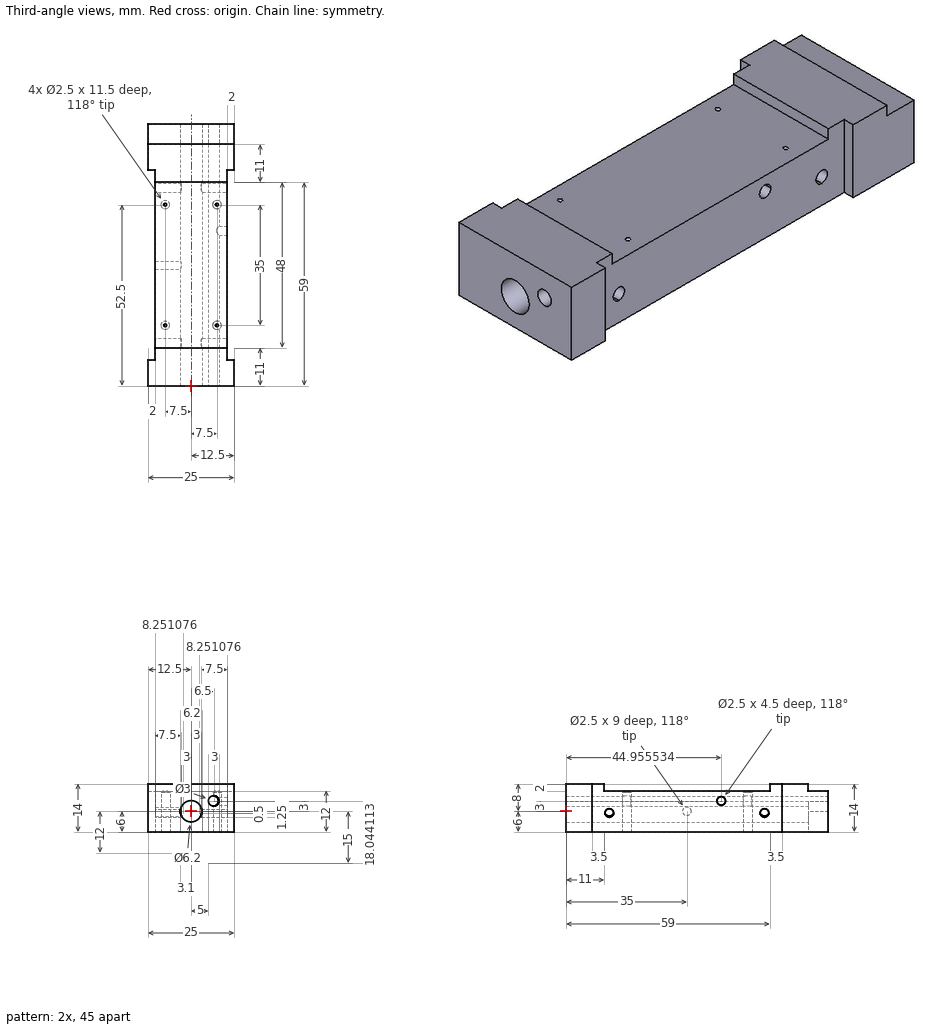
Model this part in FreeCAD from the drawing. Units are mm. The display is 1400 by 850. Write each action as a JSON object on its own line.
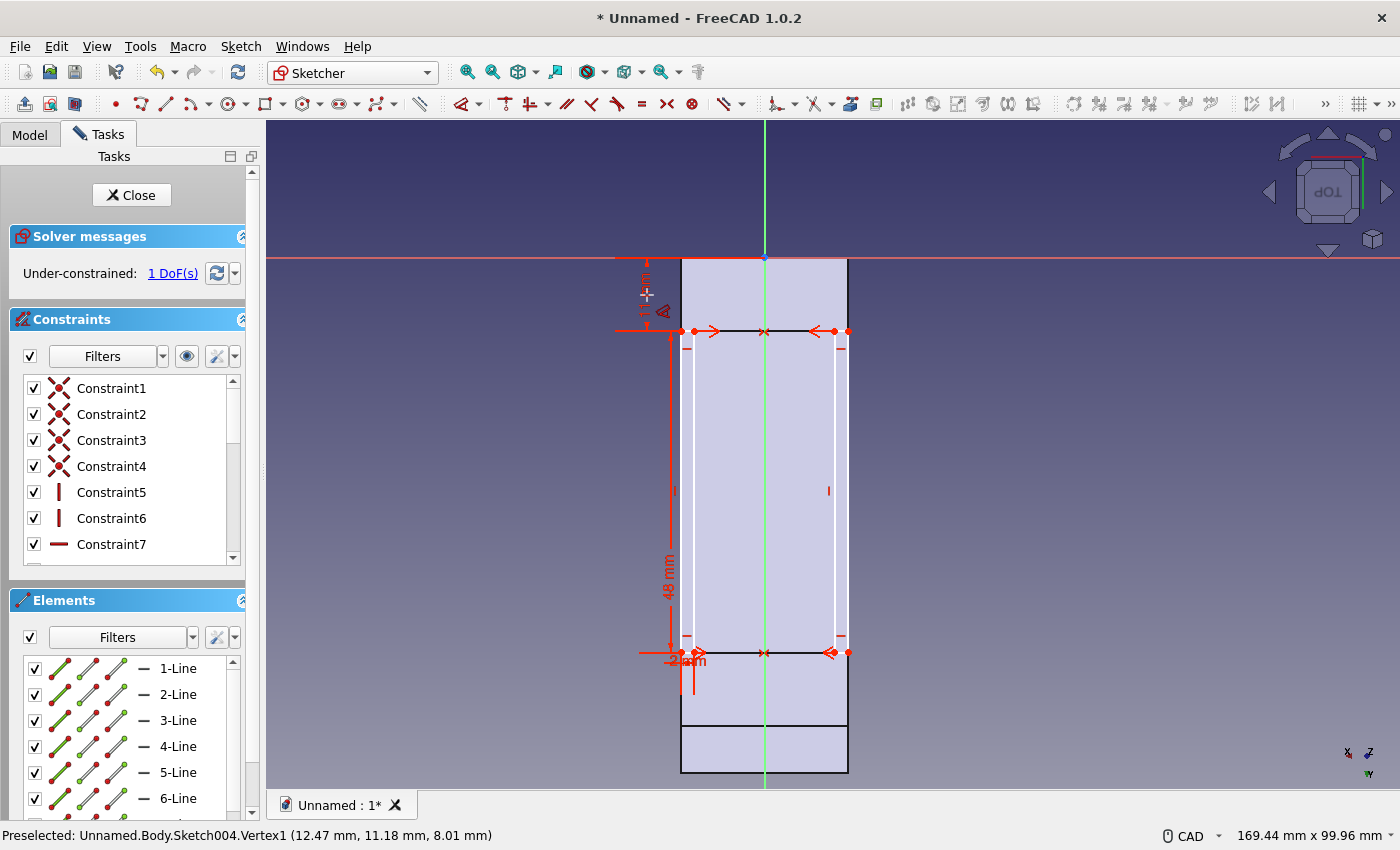
{"action": "left_click", "coordinate": [681, 331]}
{"action": "left_click", "coordinate": [723, 224]}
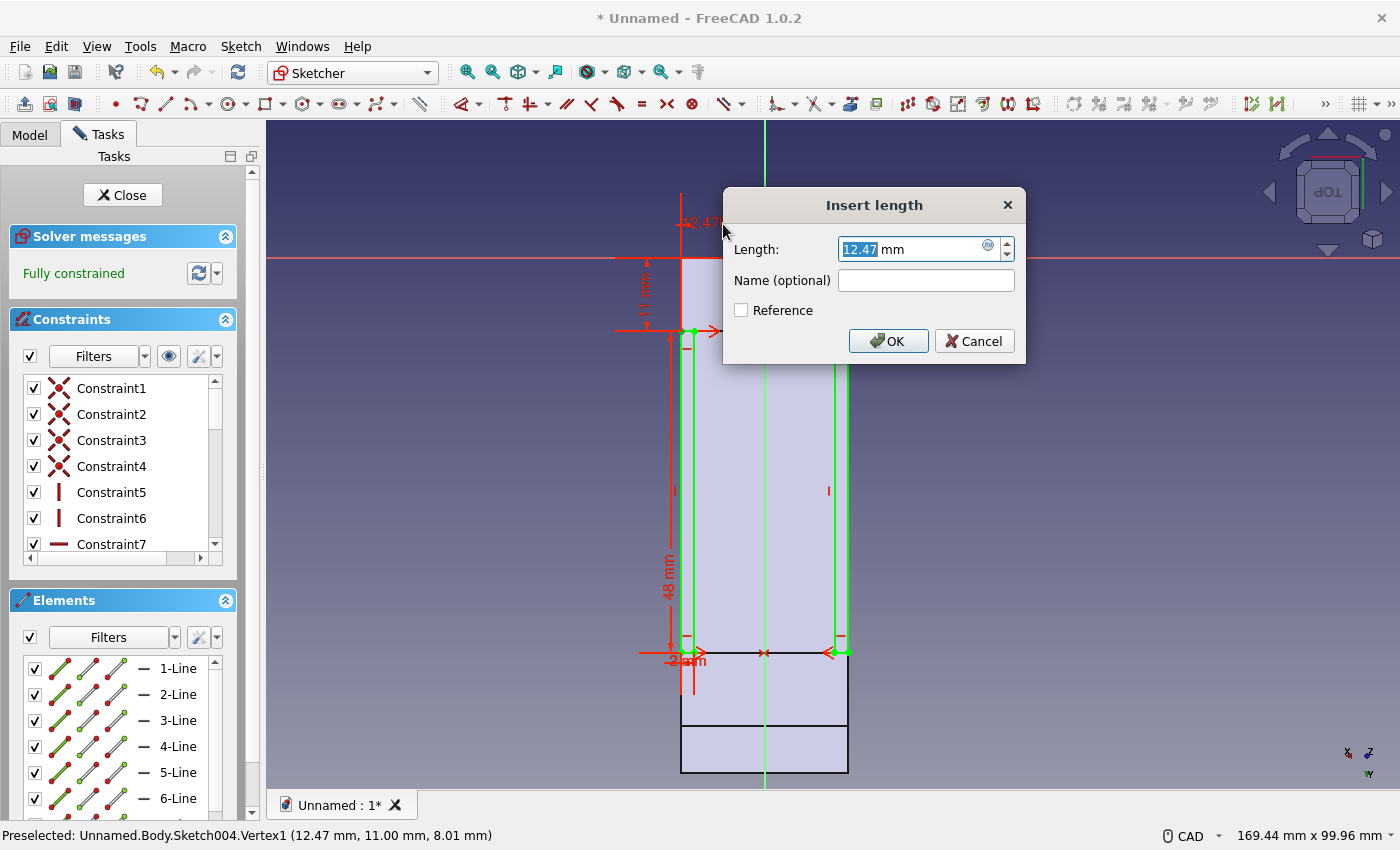
{"action": "type", "text": "12.5"}
{"action": "key", "text": "Return"}
{"action": "key", "text": "Escape"}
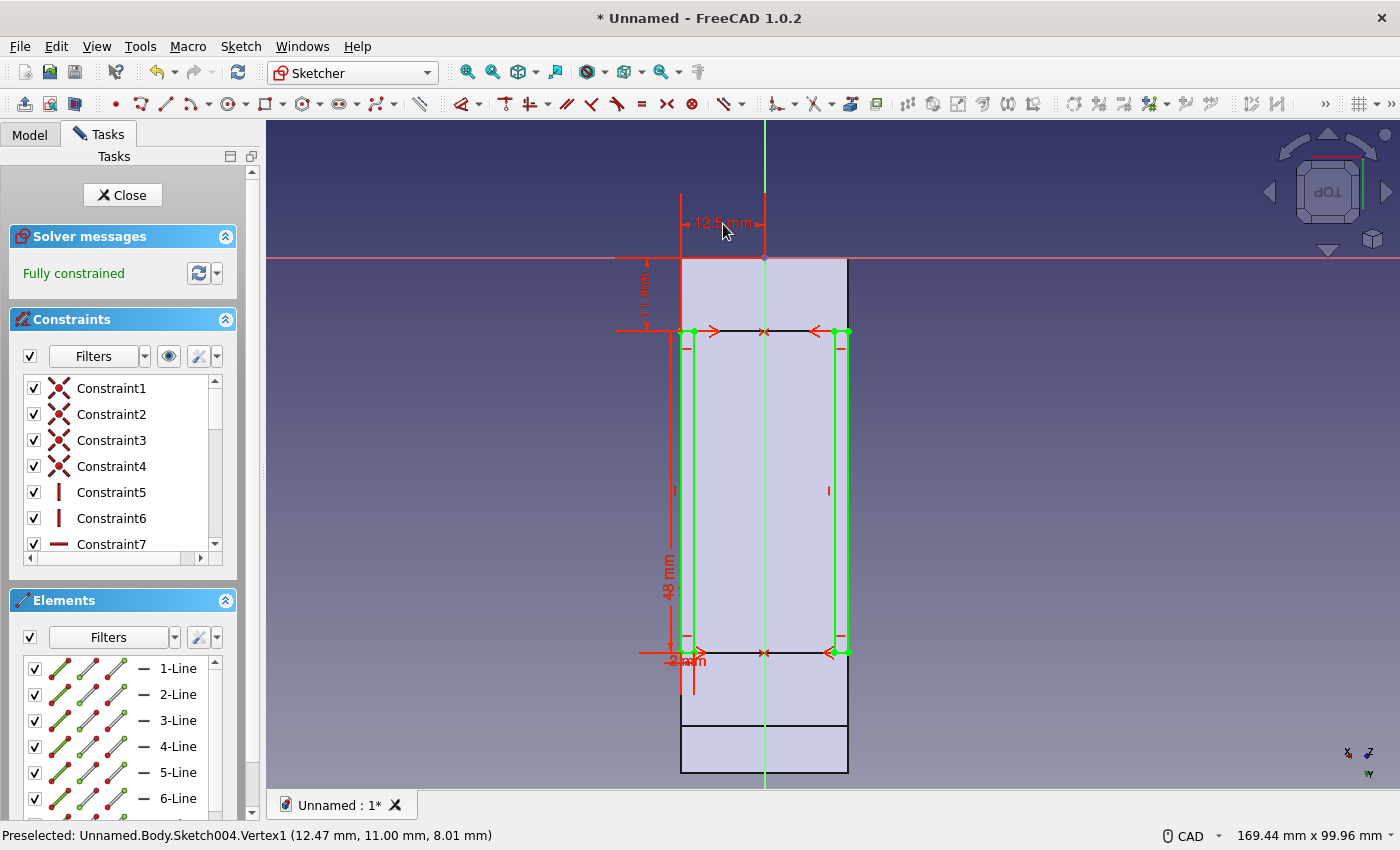
{"action": "left_click", "coordinate": [123, 195]}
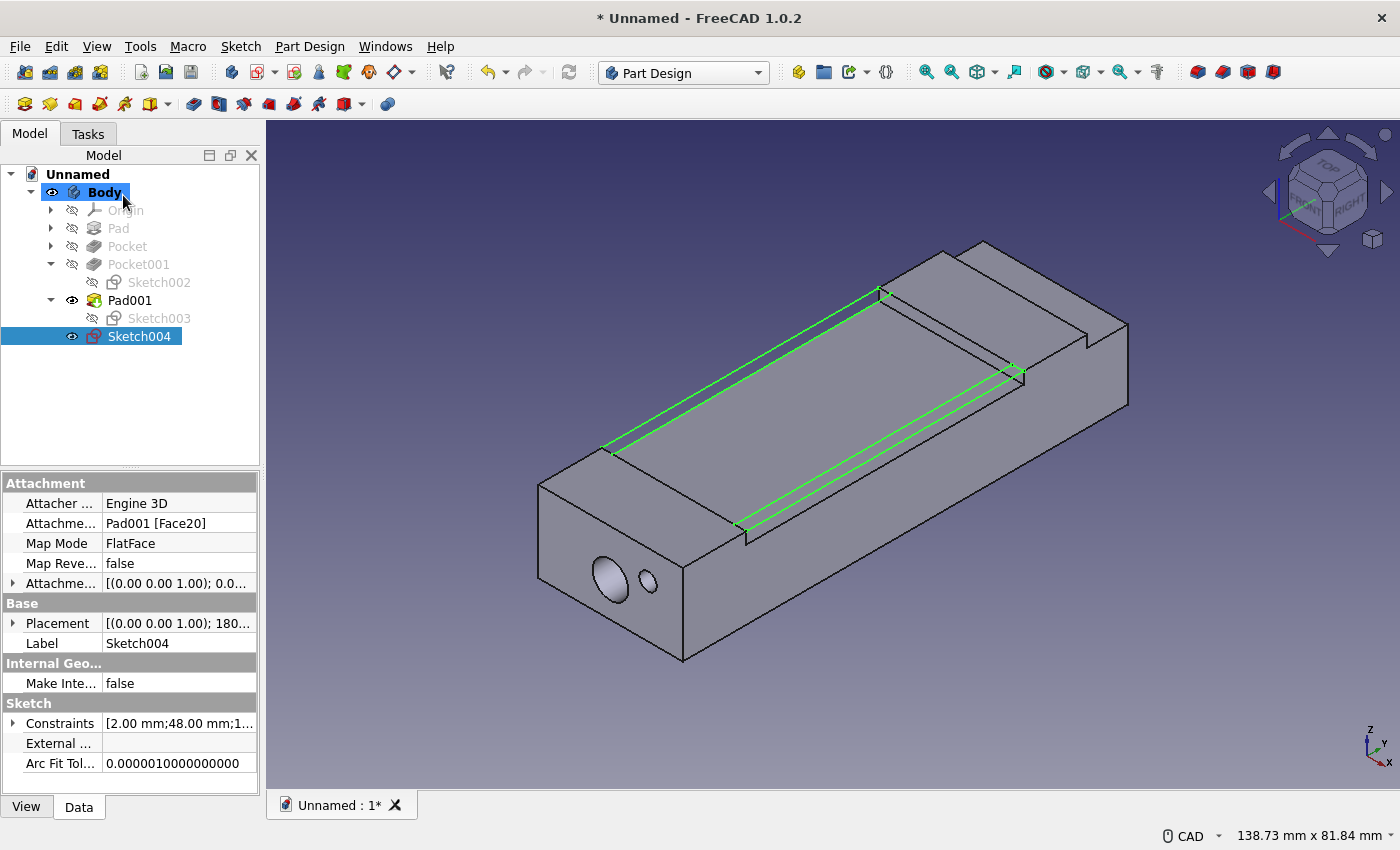
{"action": "left_click", "coordinate": [194, 104]}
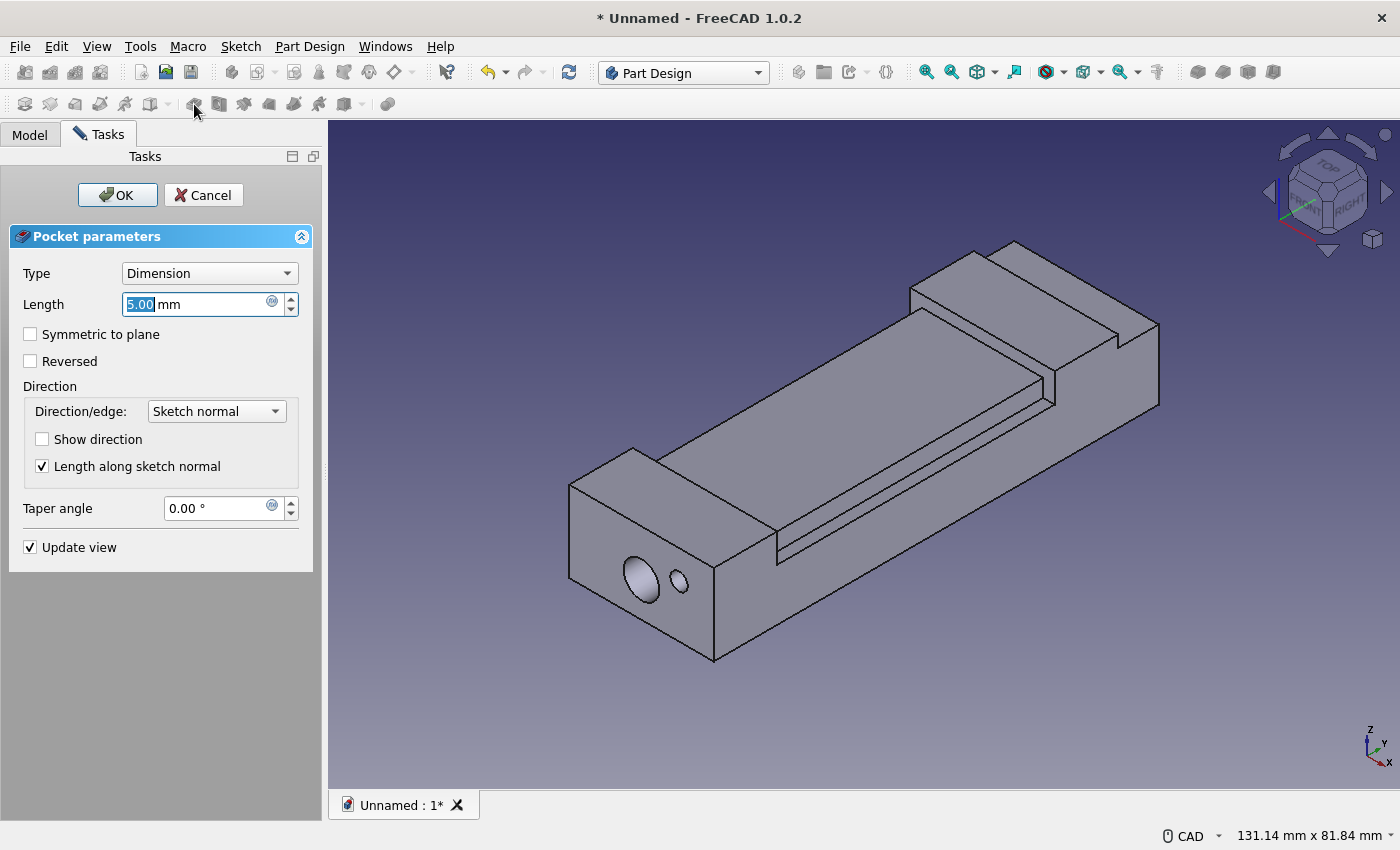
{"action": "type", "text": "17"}
{"action": "key", "text": "Tab"}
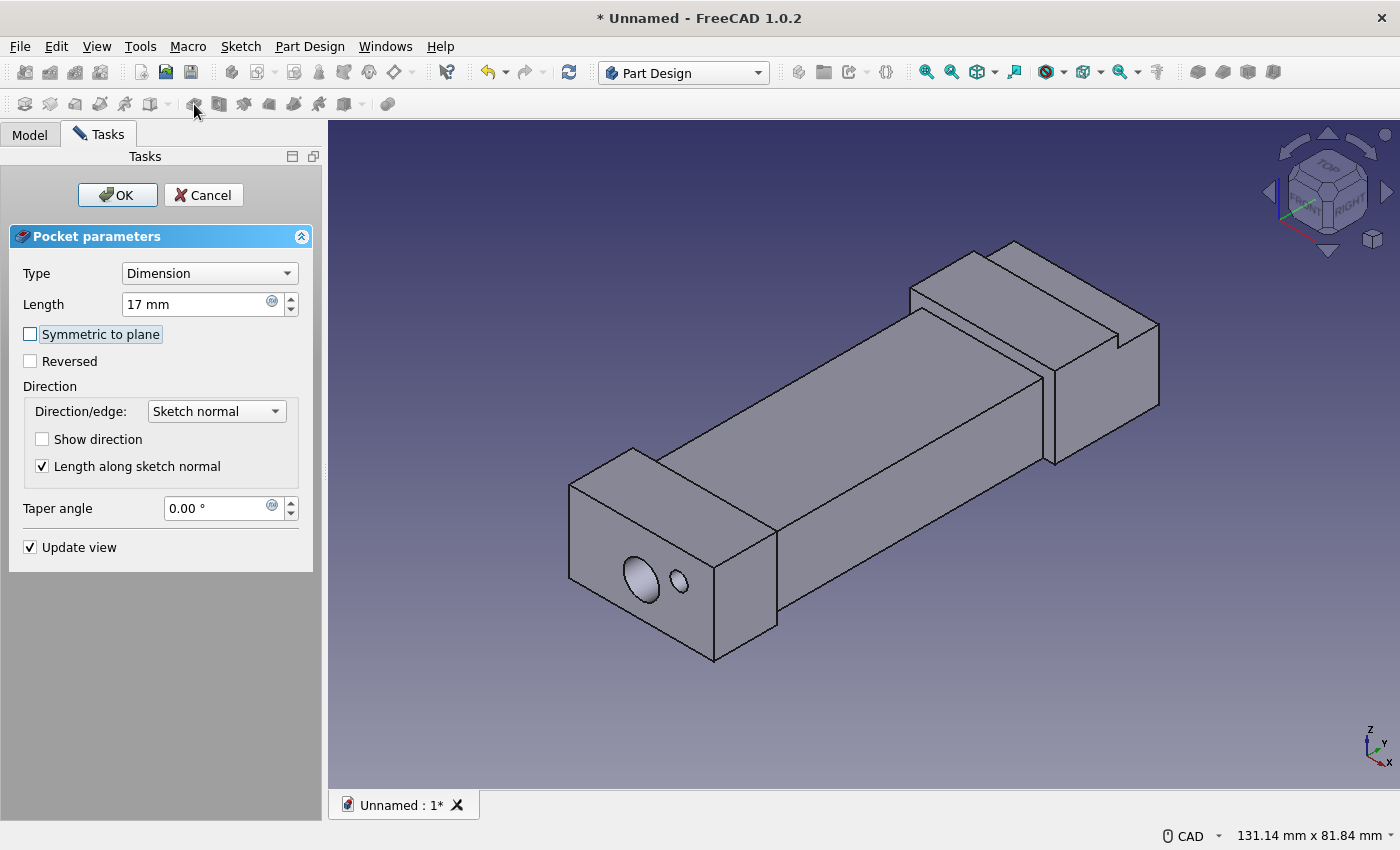
{"action": "left_click", "coordinate": [118, 195]}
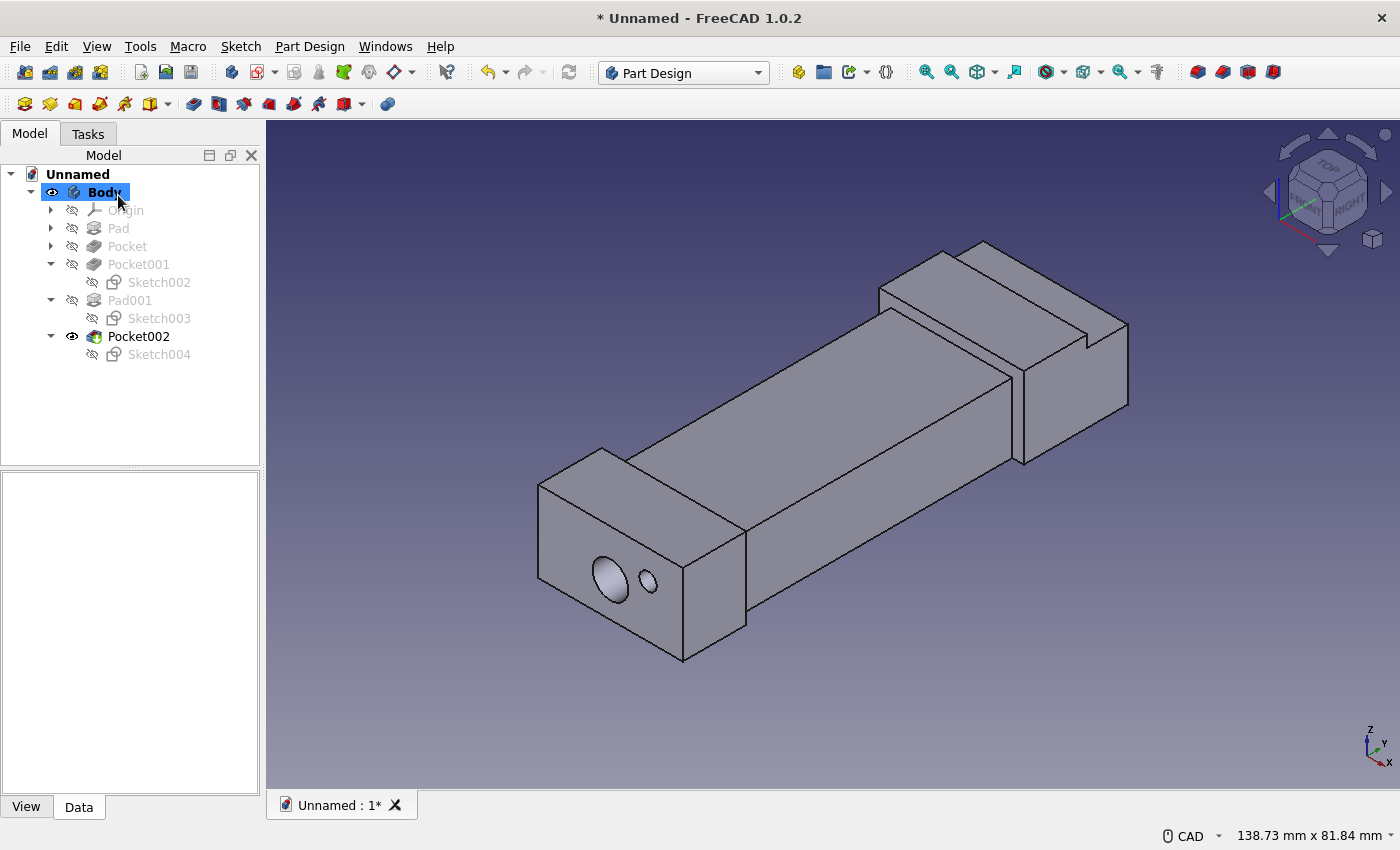
{"action": "left_click", "coordinate": [51, 210]}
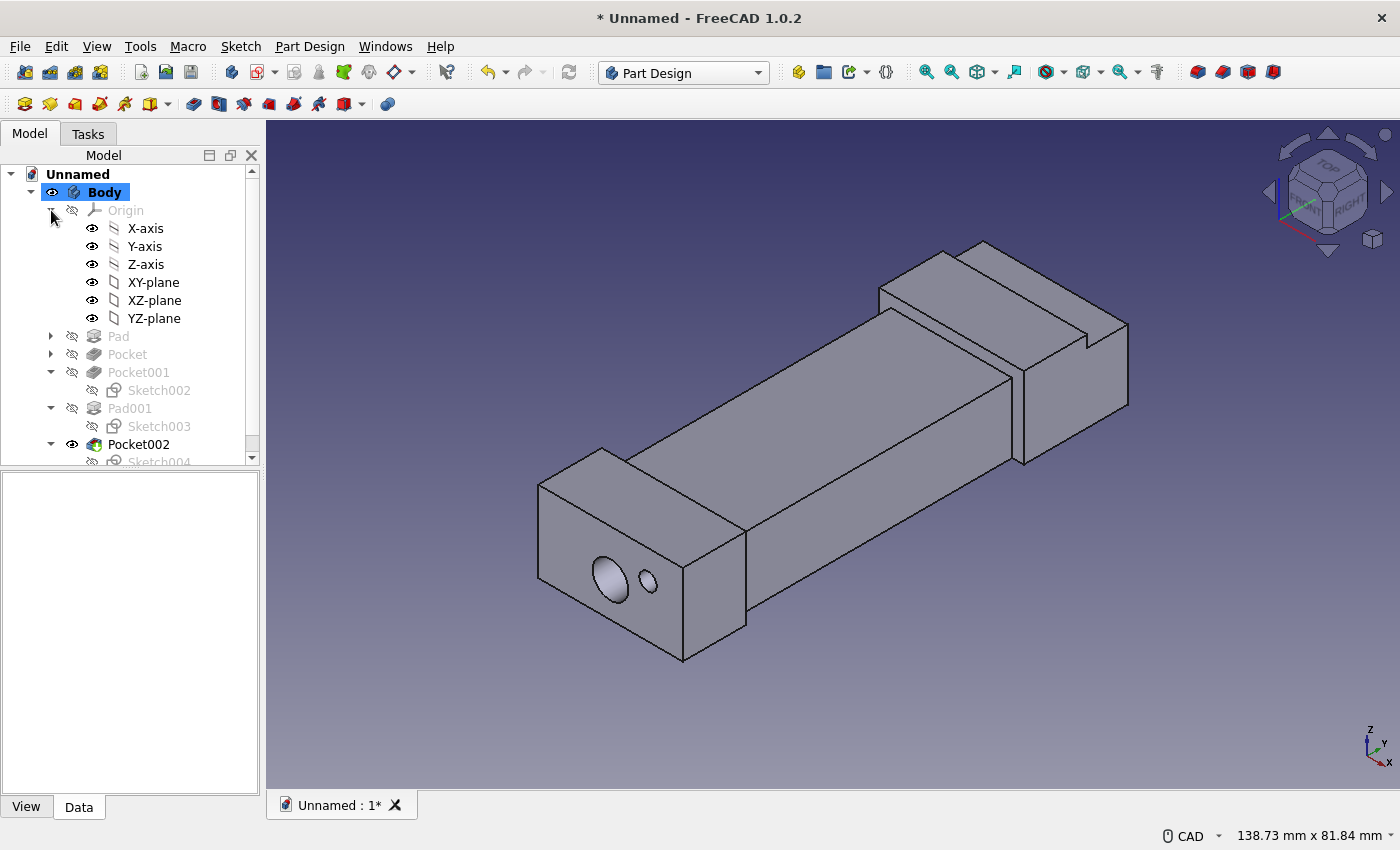
{"action": "left_click", "coordinate": [137, 300]}